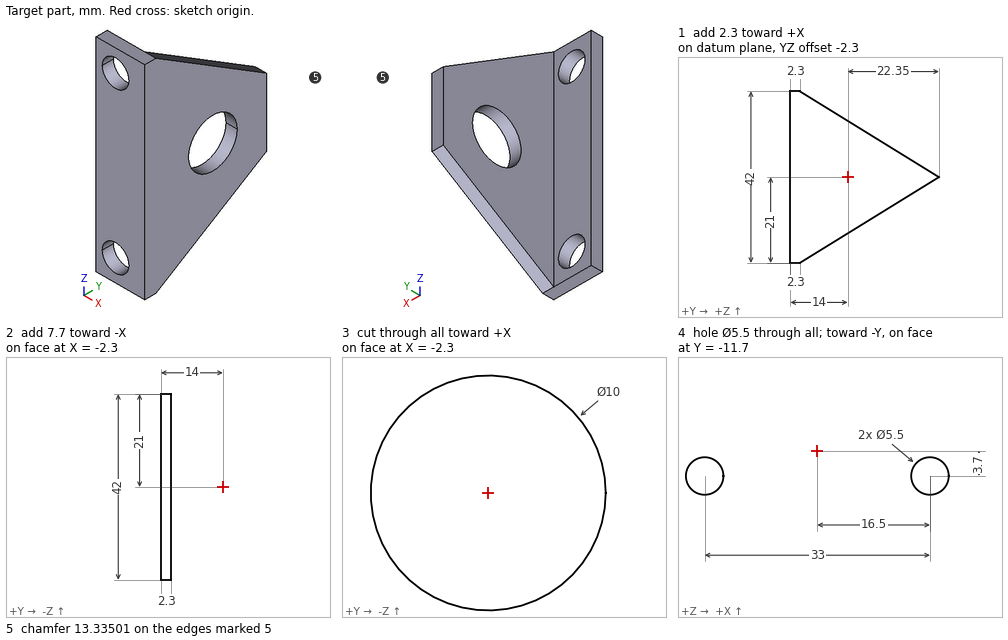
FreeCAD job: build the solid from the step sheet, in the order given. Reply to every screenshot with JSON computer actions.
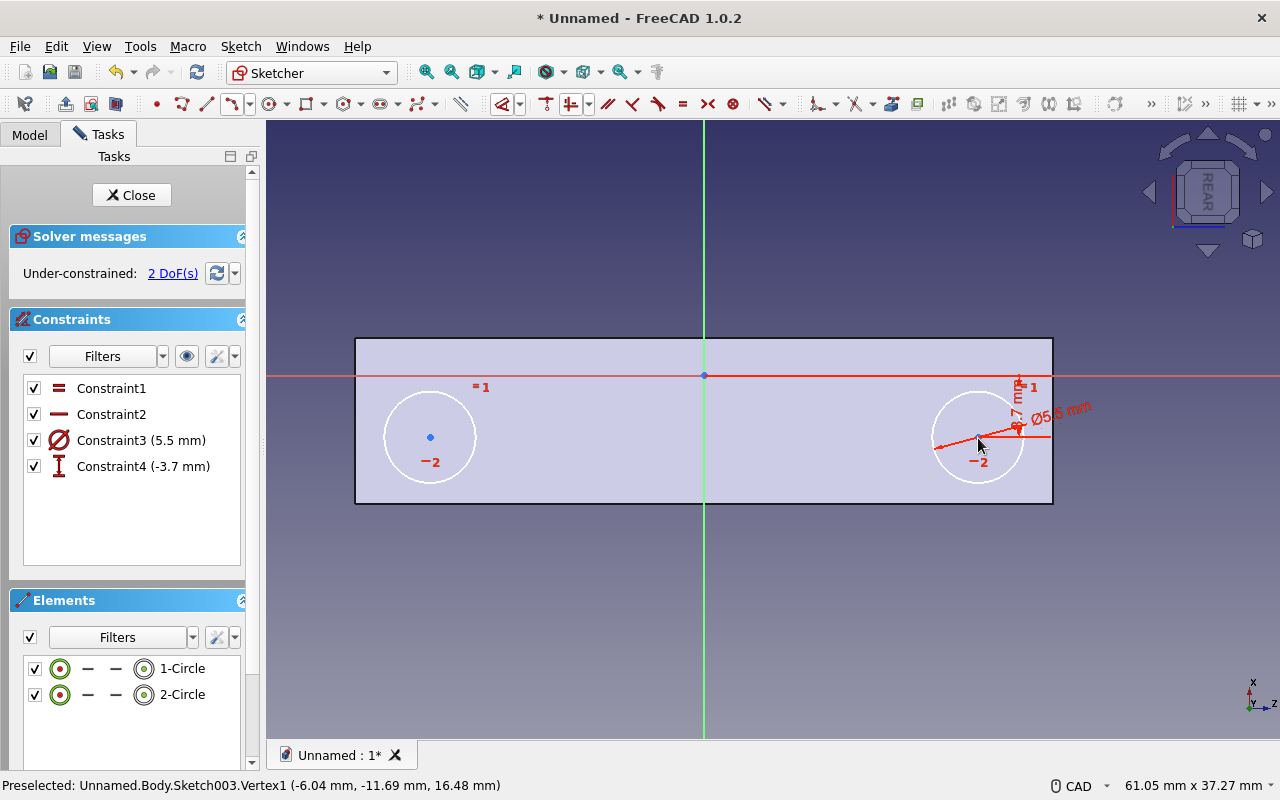
{"action": "left_click", "coordinate": [978, 437]}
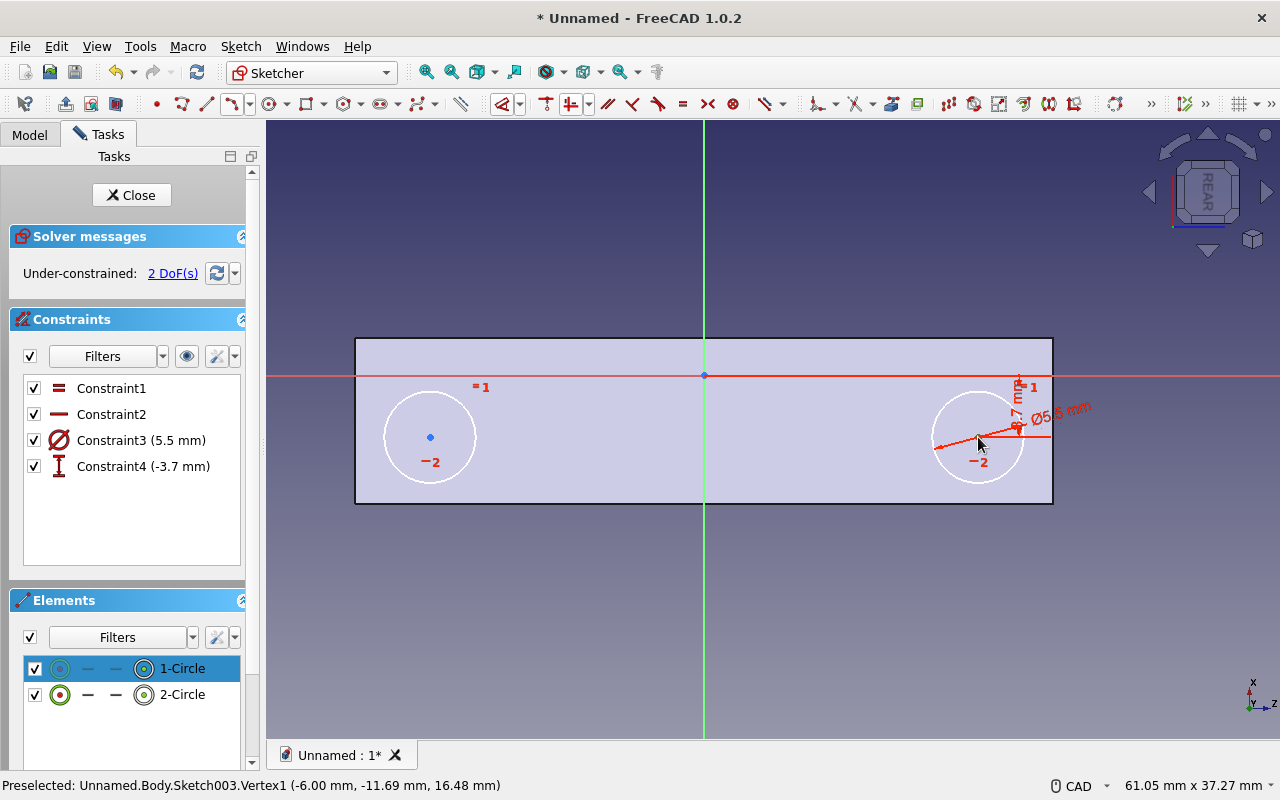
{"action": "left_click", "coordinate": [430, 437]}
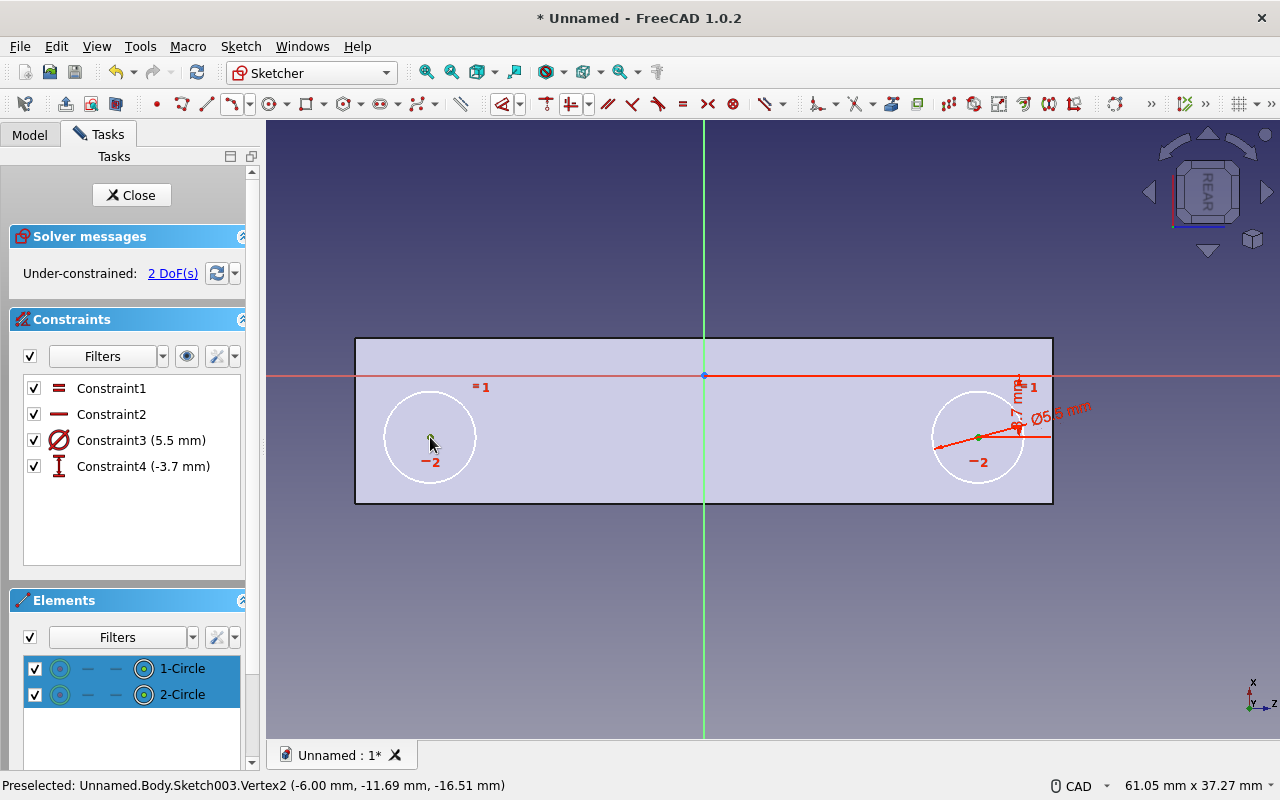
{"action": "key", "text": "l"}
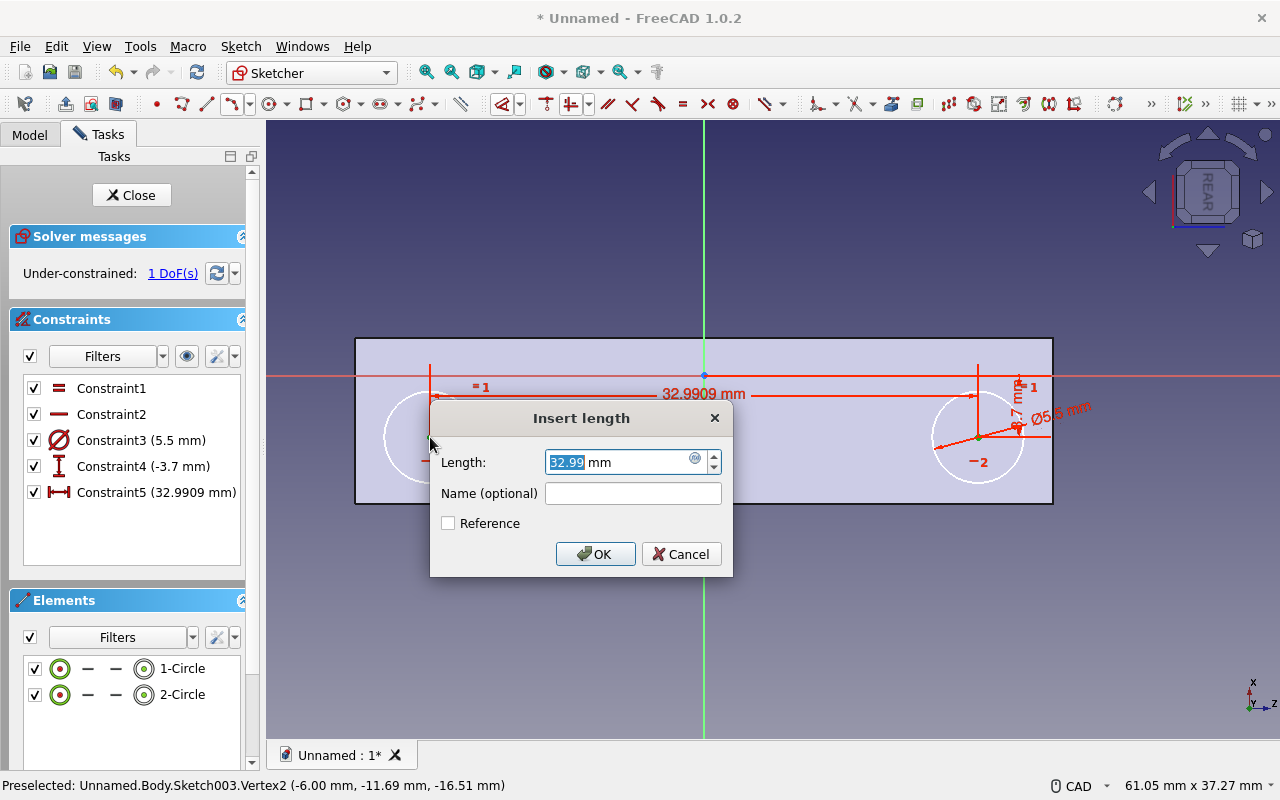
{"action": "type", "text": "33"}
{"action": "key", "text": "Return"}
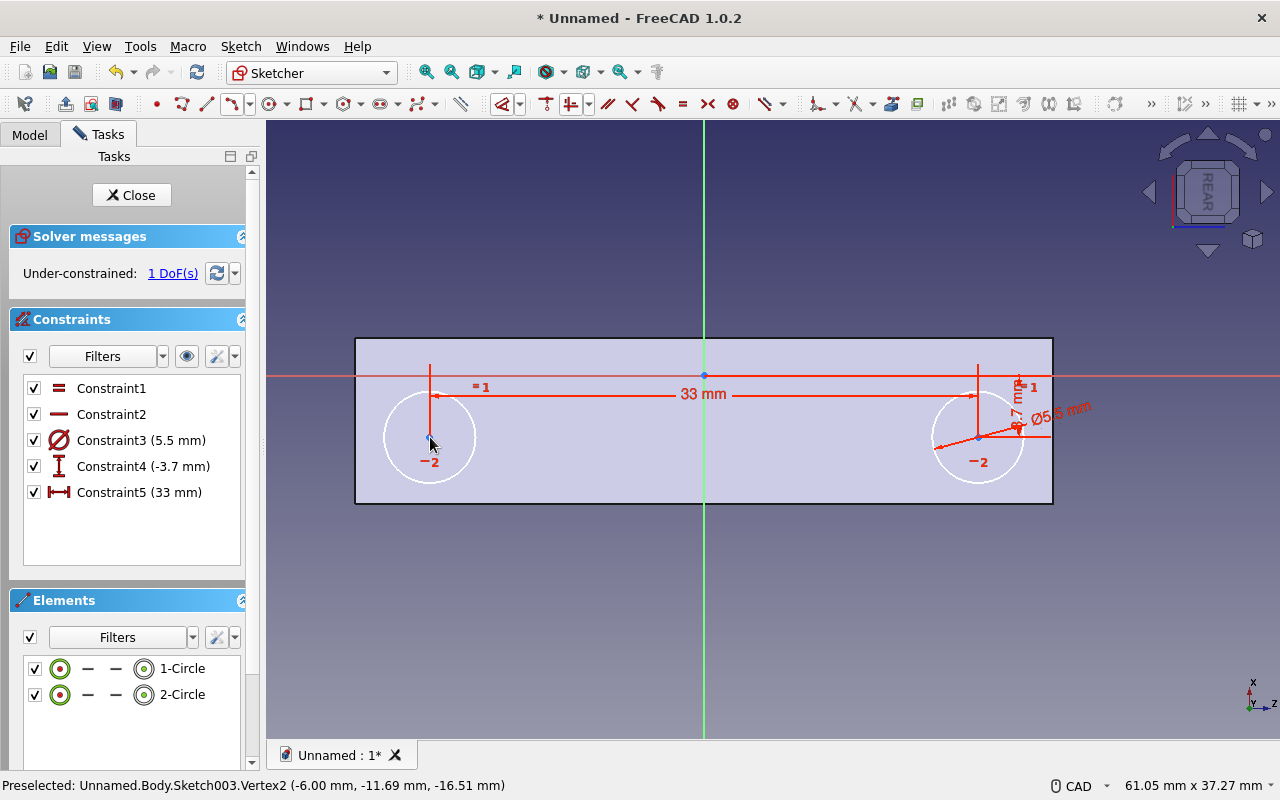
{"action": "left_click", "coordinate": [978, 437]}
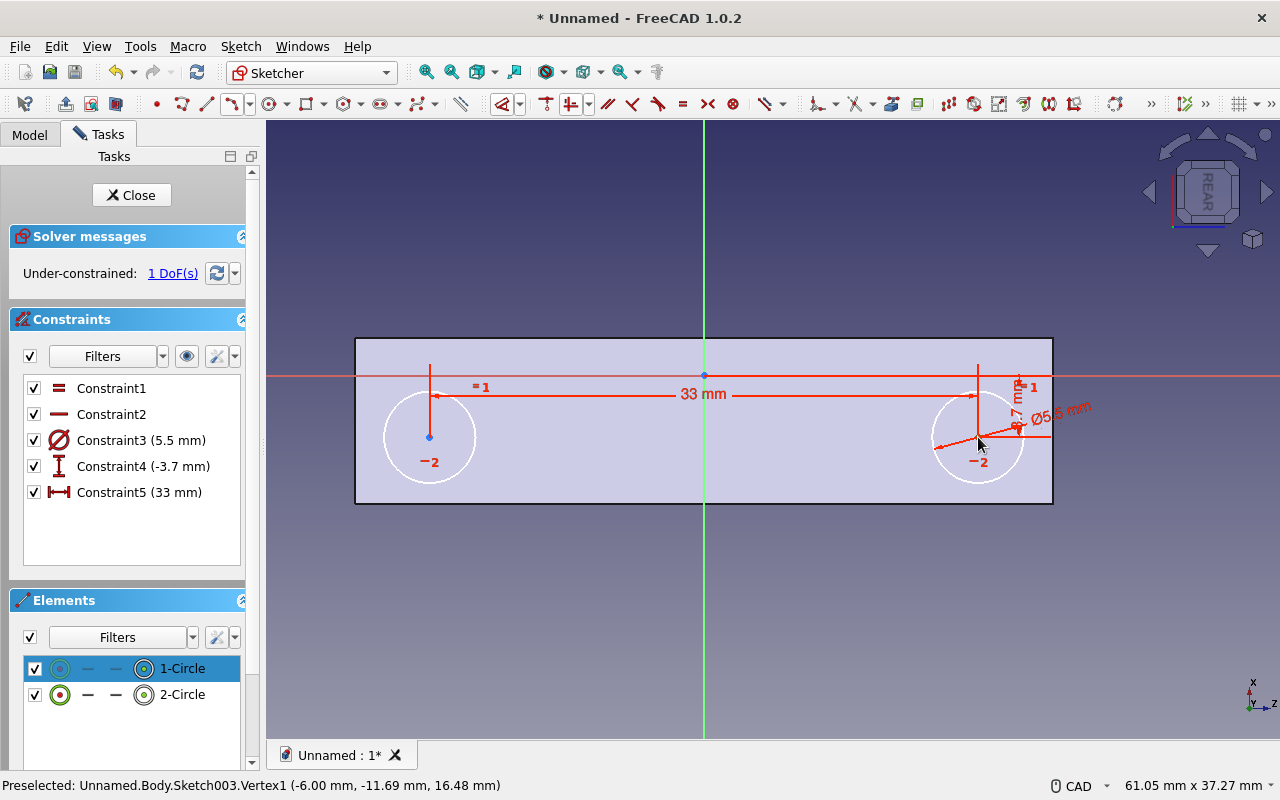
{"action": "key", "text": "l"}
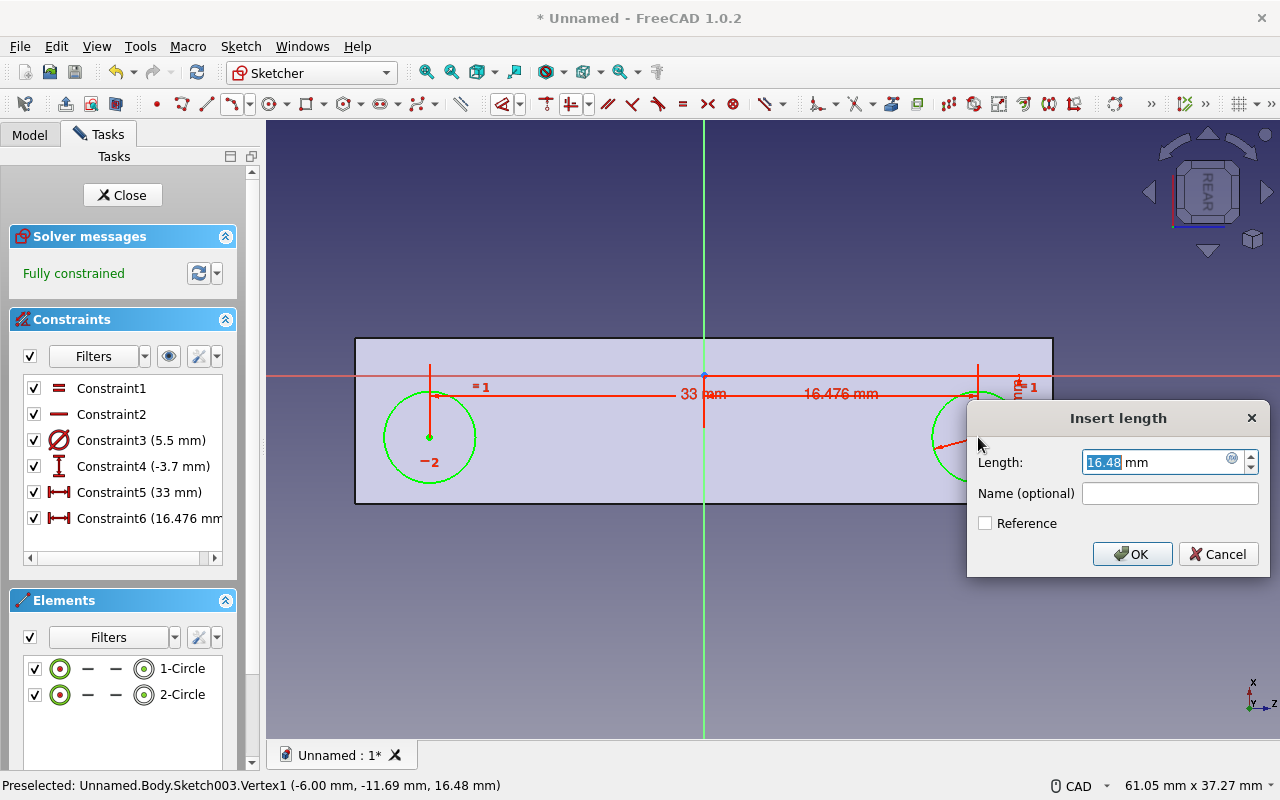
{"action": "type", "text": "16.5"}
{"action": "key", "text": "Return"}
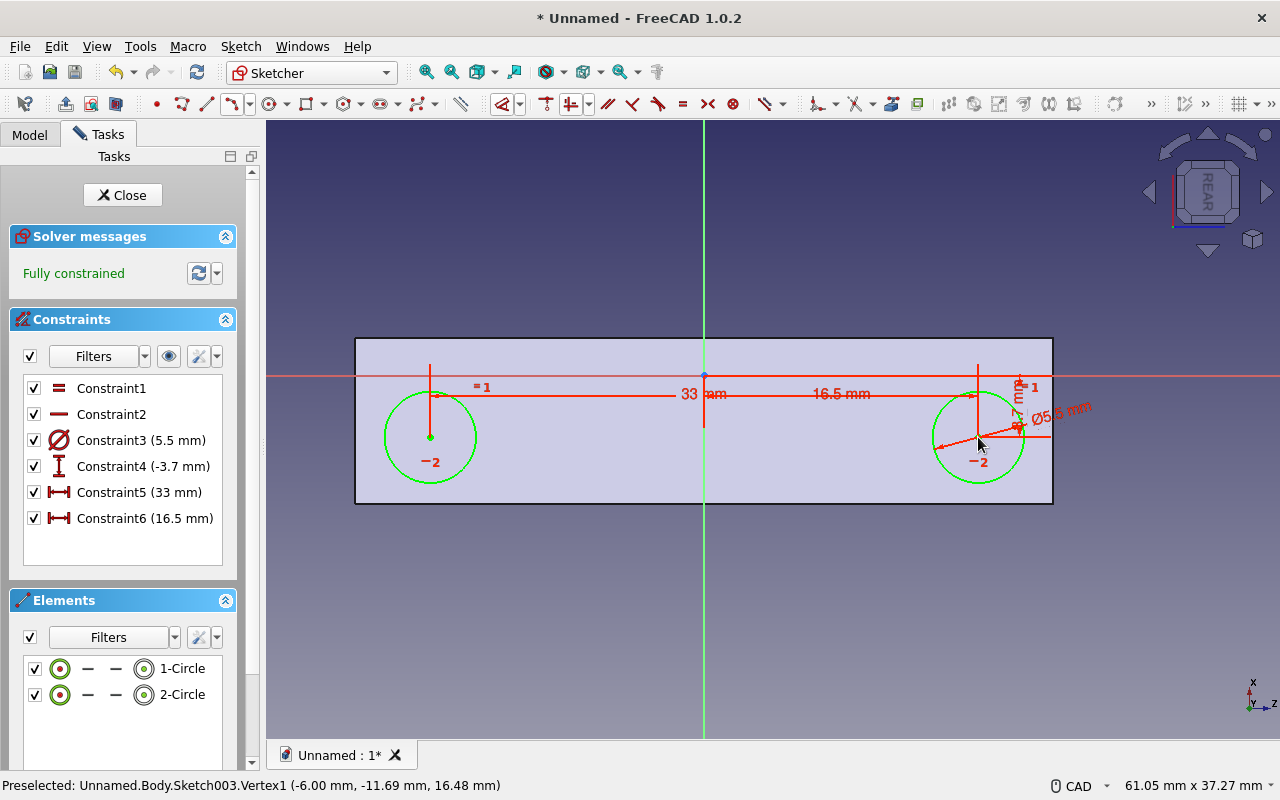
{"action": "left_click", "coordinate": [123, 195]}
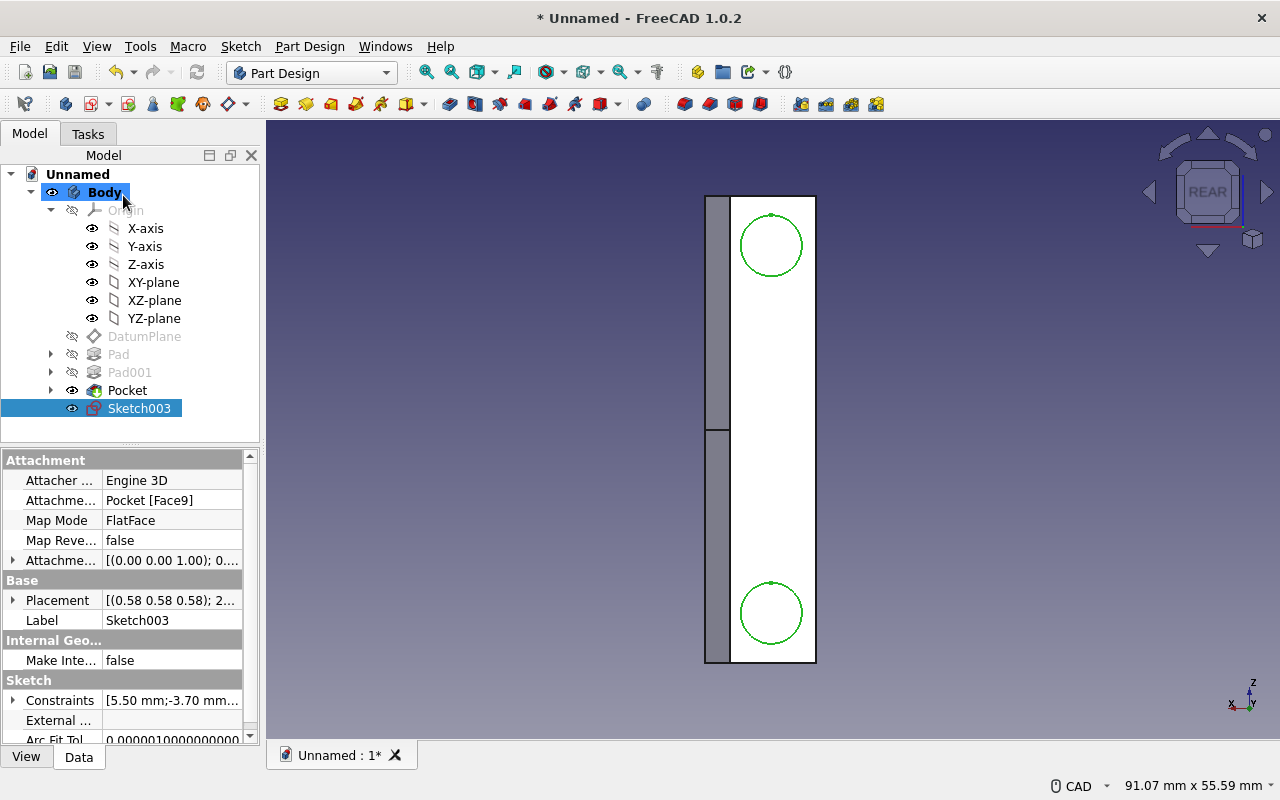
{"action": "left_click", "coordinate": [475, 104]}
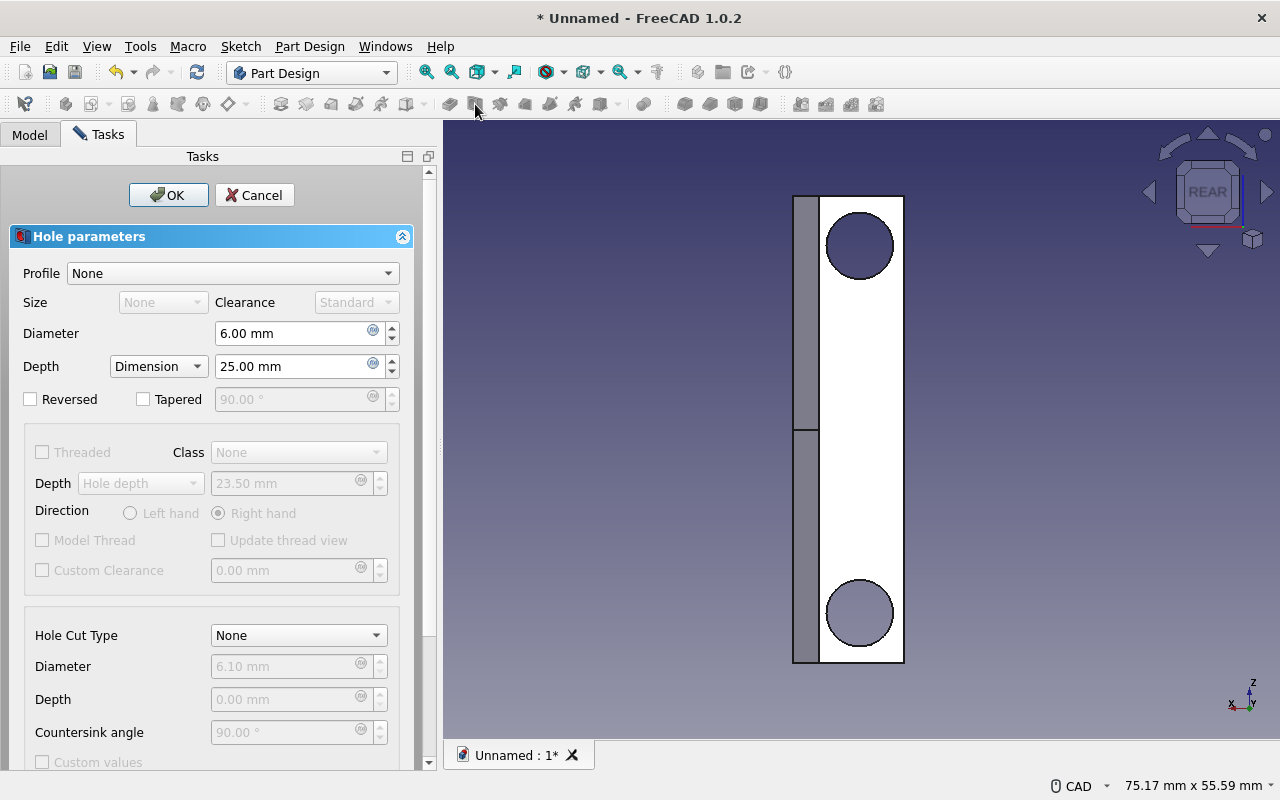
{"action": "triple_click", "coordinate": [300, 334]}